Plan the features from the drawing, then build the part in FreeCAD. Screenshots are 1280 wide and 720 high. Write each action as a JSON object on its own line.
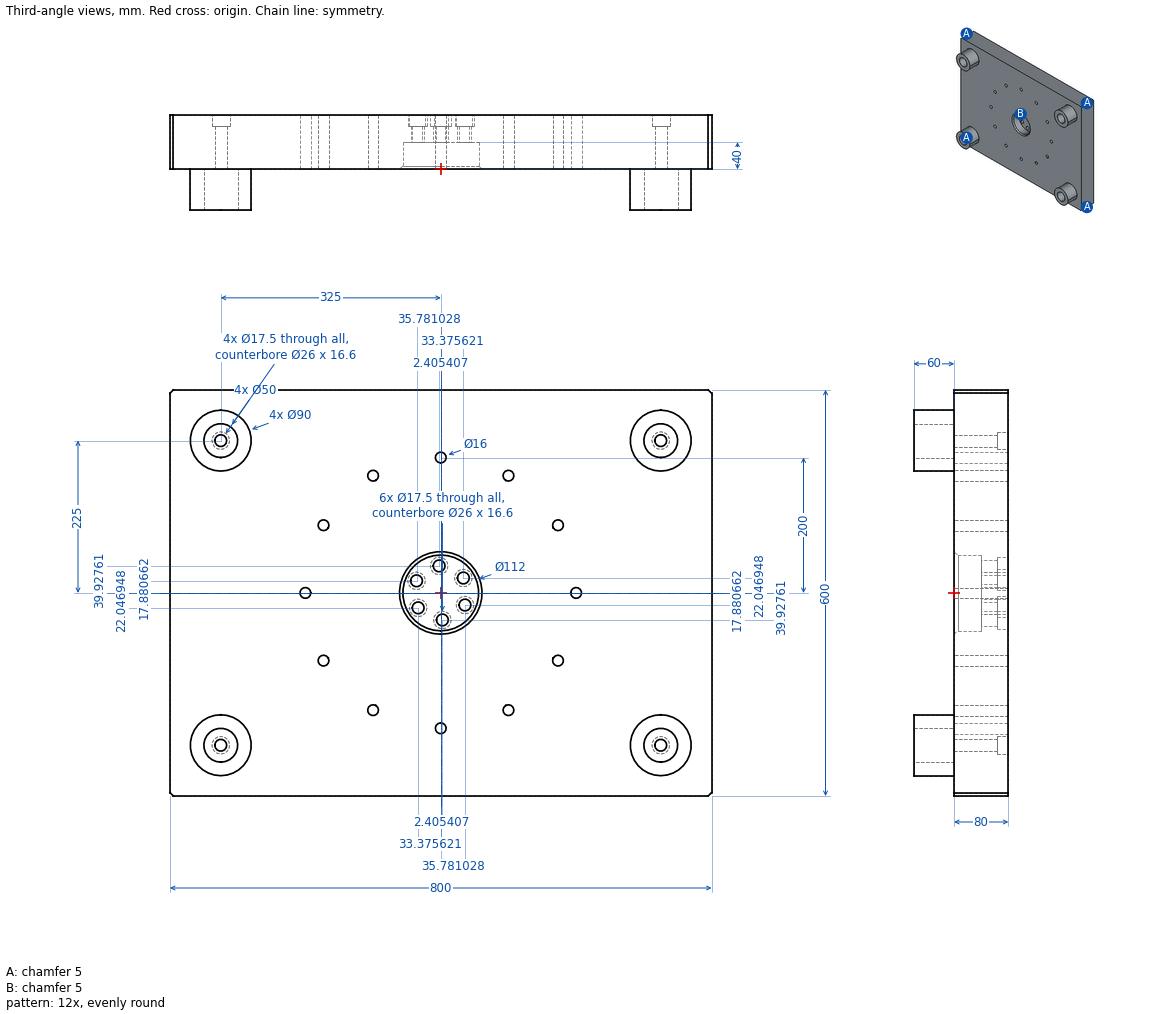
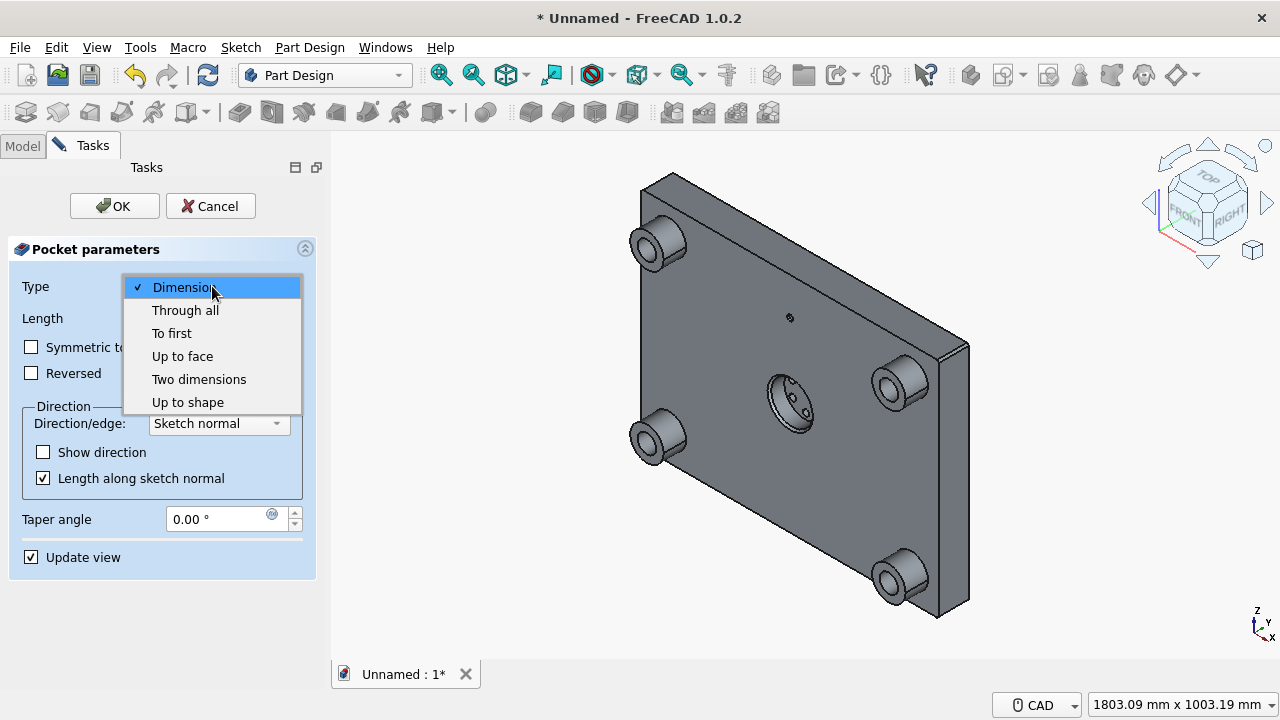
{"action": "left_click", "coordinate": [212, 310]}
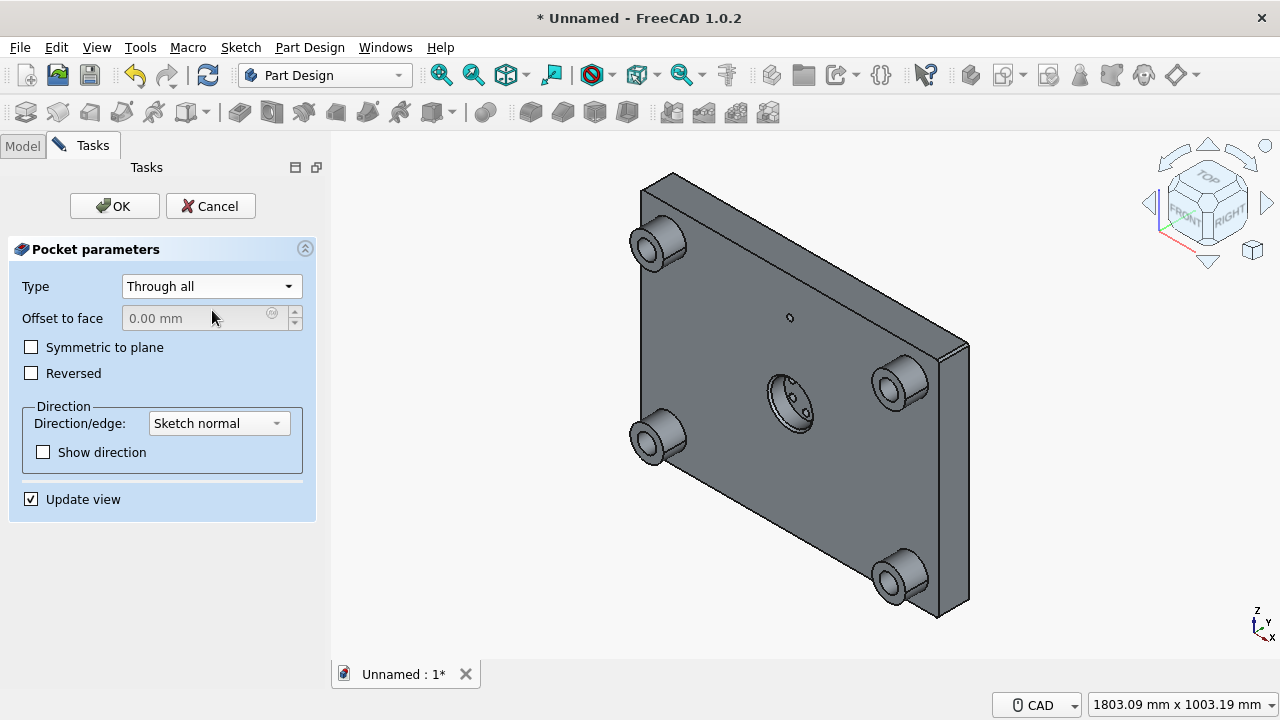
{"action": "left_click", "coordinate": [115, 206]}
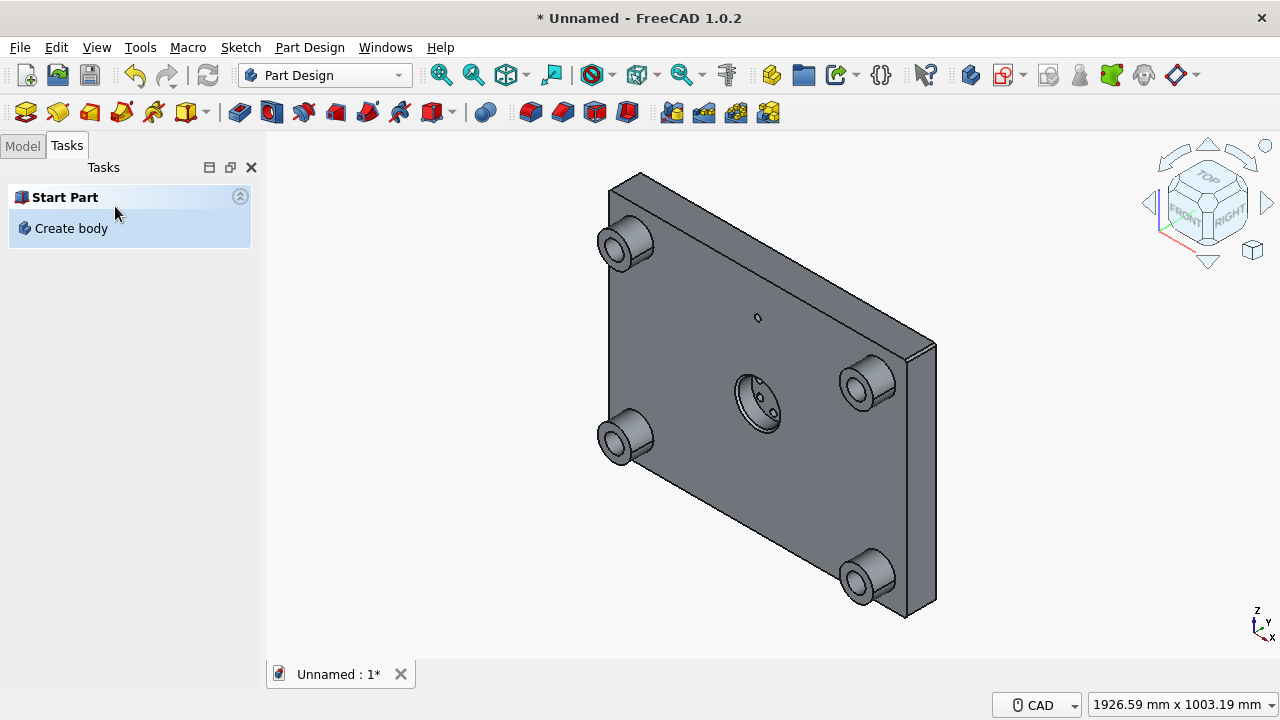
{"action": "left_click", "coordinate": [23, 145]}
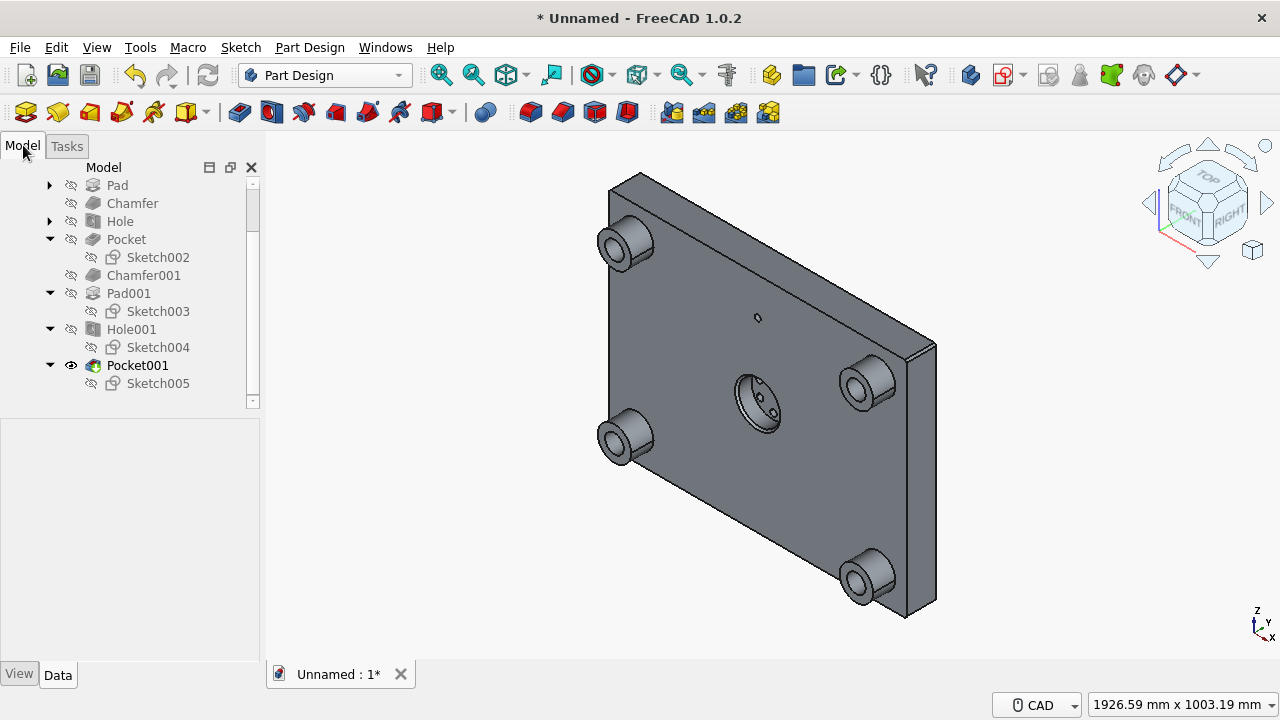
{"action": "left_click", "coordinate": [116, 365]}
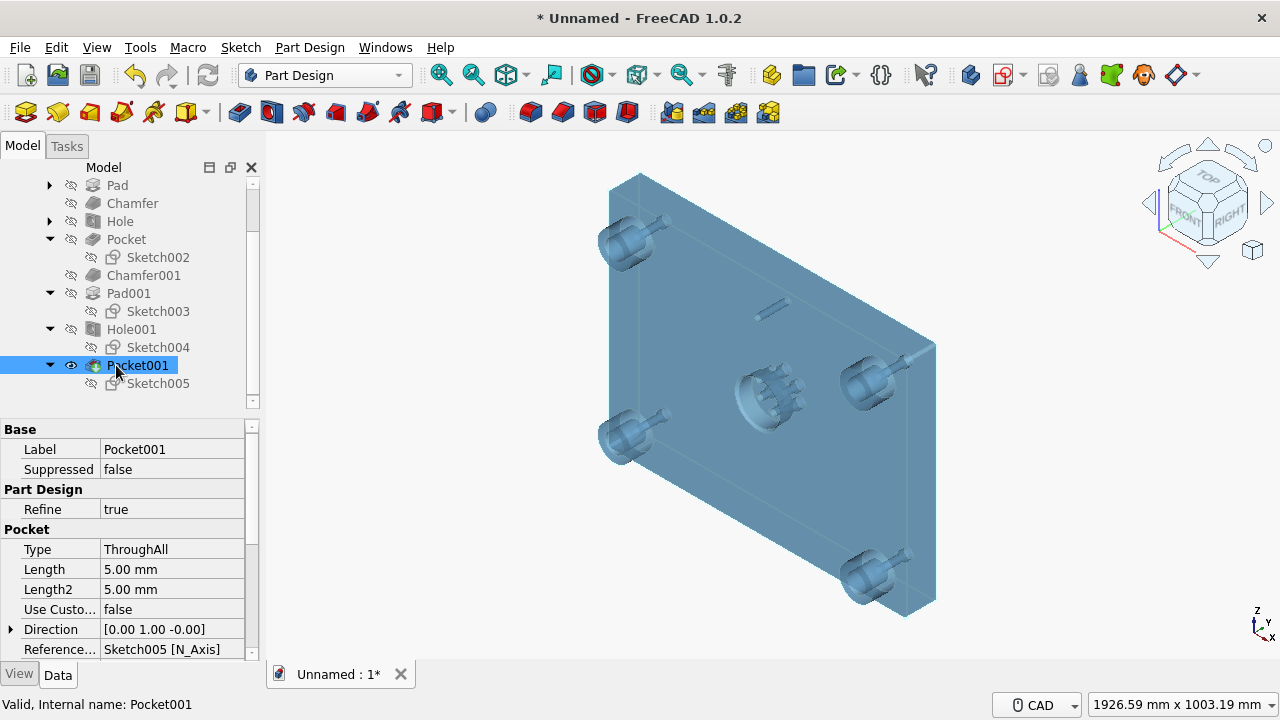
{"action": "left_click", "coordinate": [736, 112]}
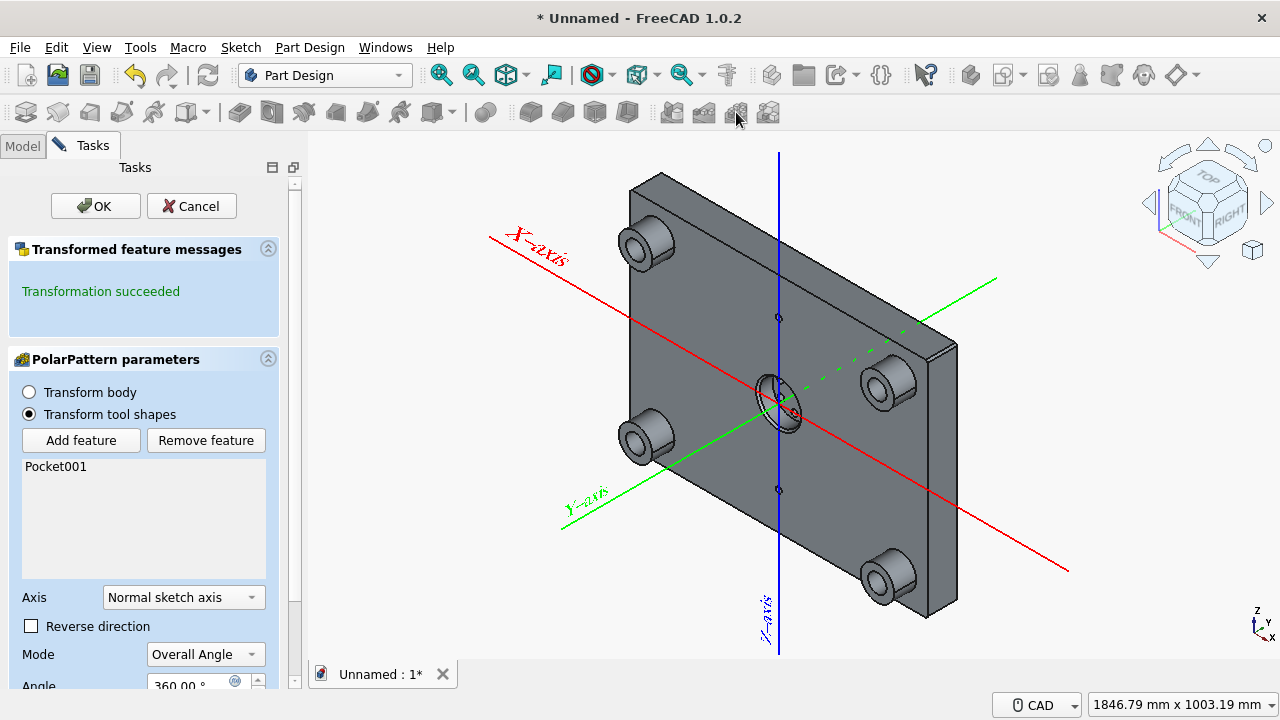
{"action": "left_click", "coordinate": [184, 598]}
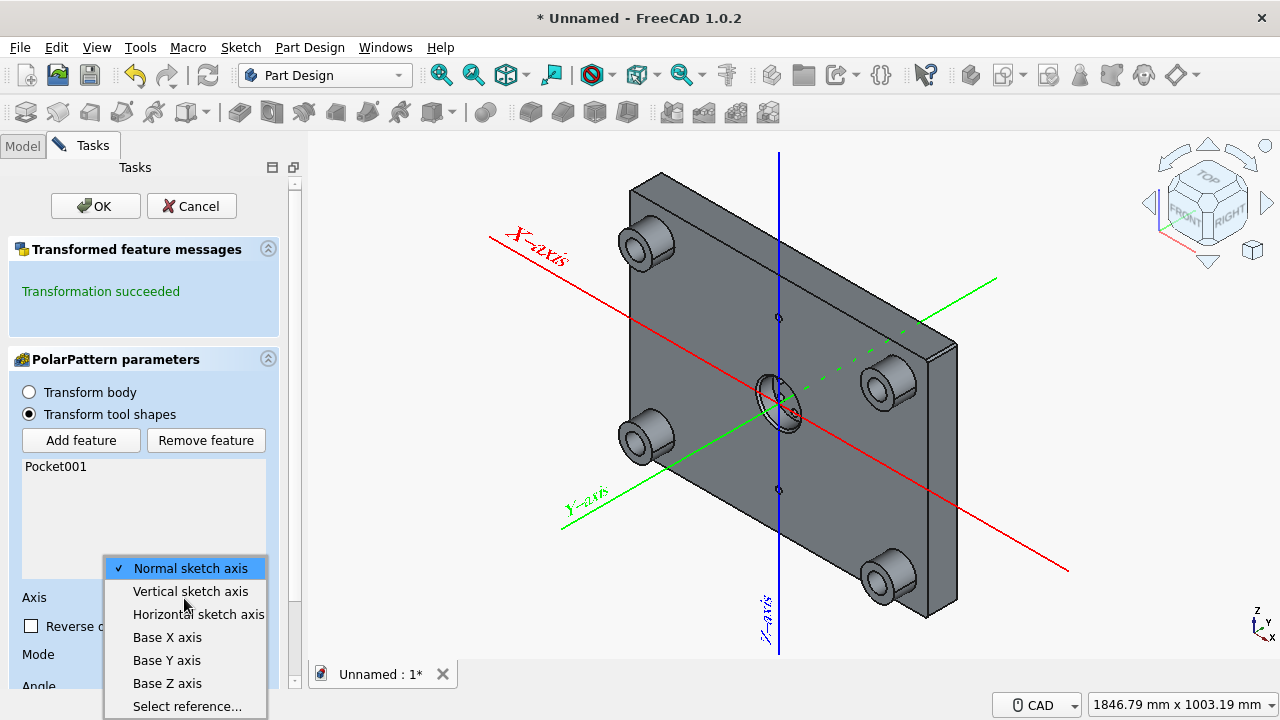
{"action": "left_click", "coordinate": [184, 660]}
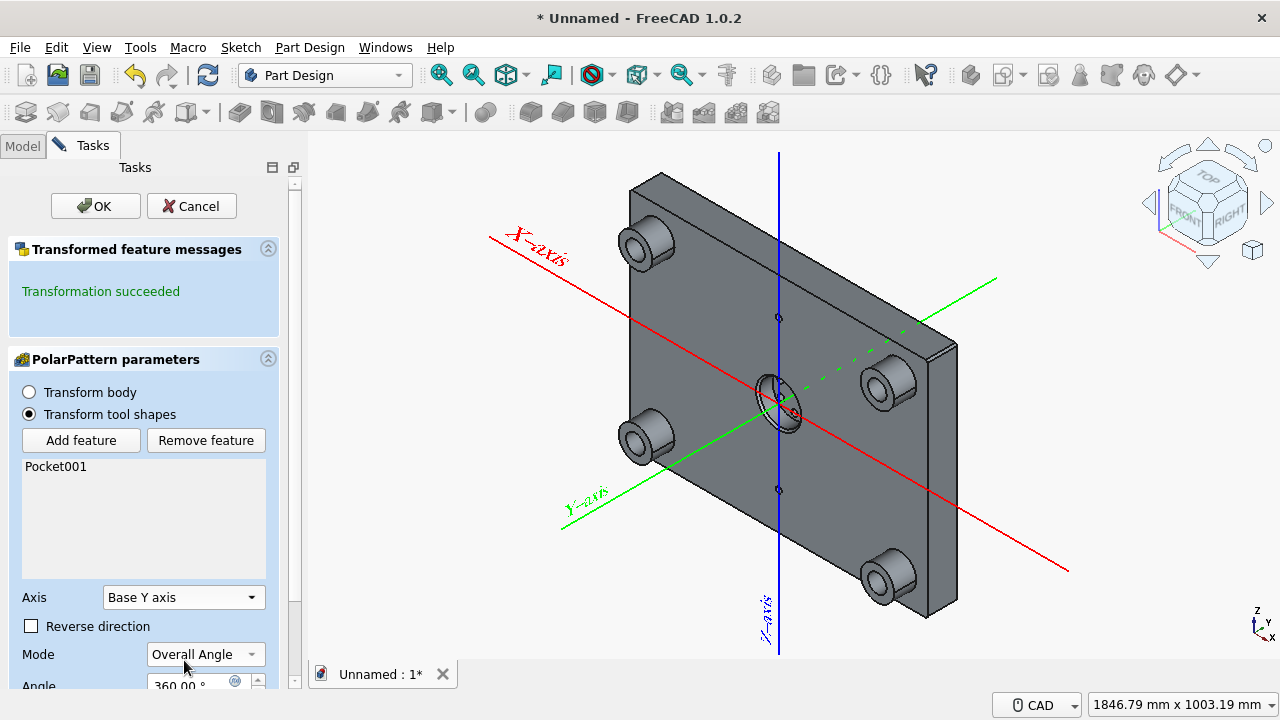
{"action": "scroll", "coordinate": [295, 432], "scroll_direction": "down", "scroll_amount": 2}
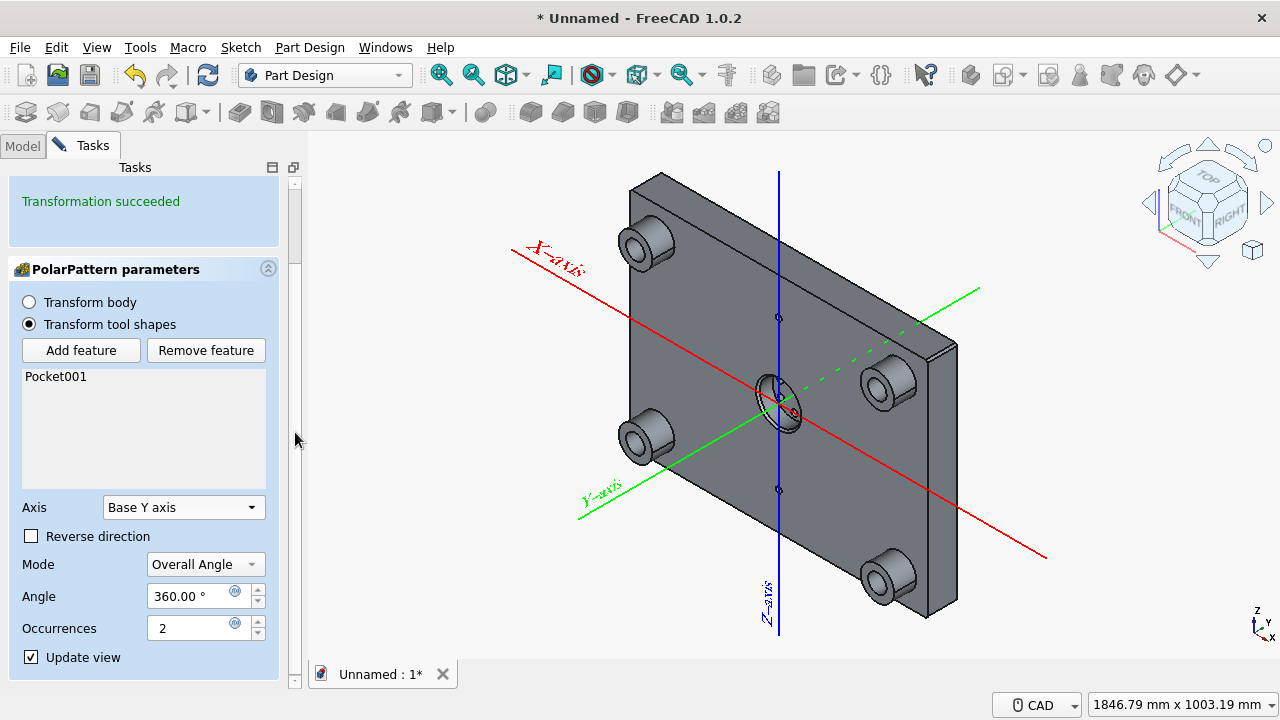
{"action": "triple_click", "coordinate": [198, 628]}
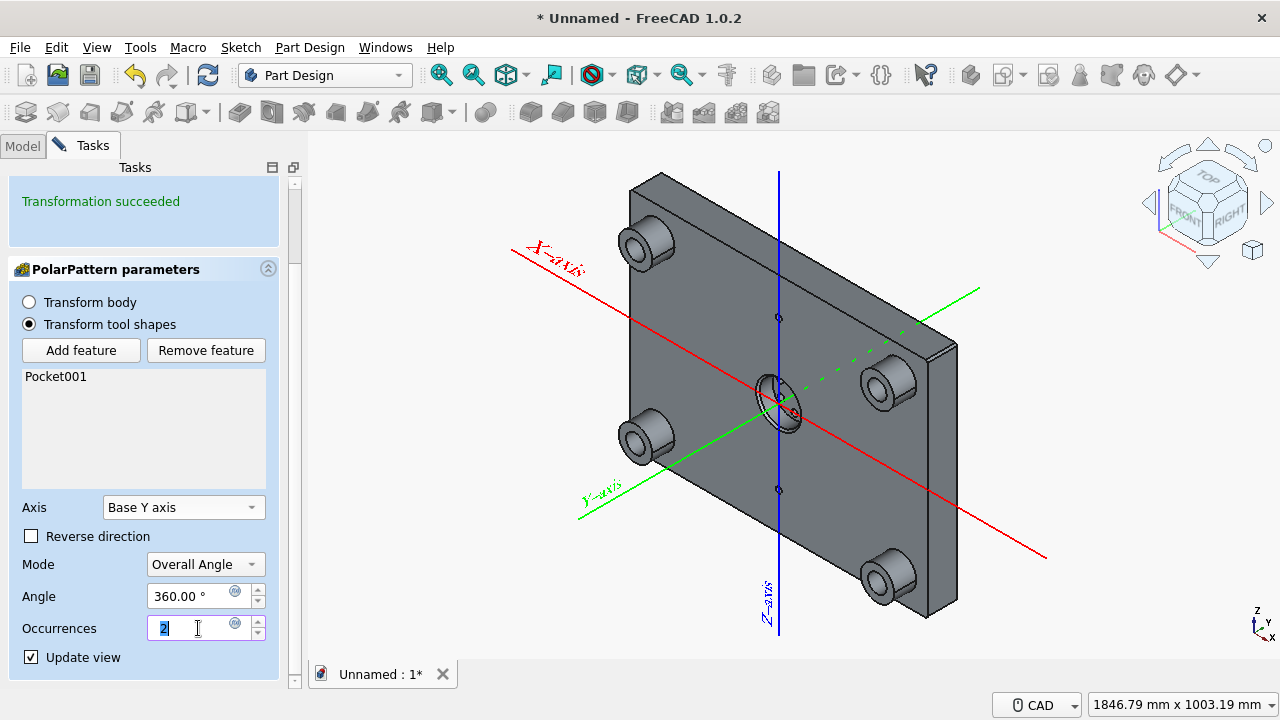
{"action": "type", "text": "12"}
{"action": "key", "text": "Tab"}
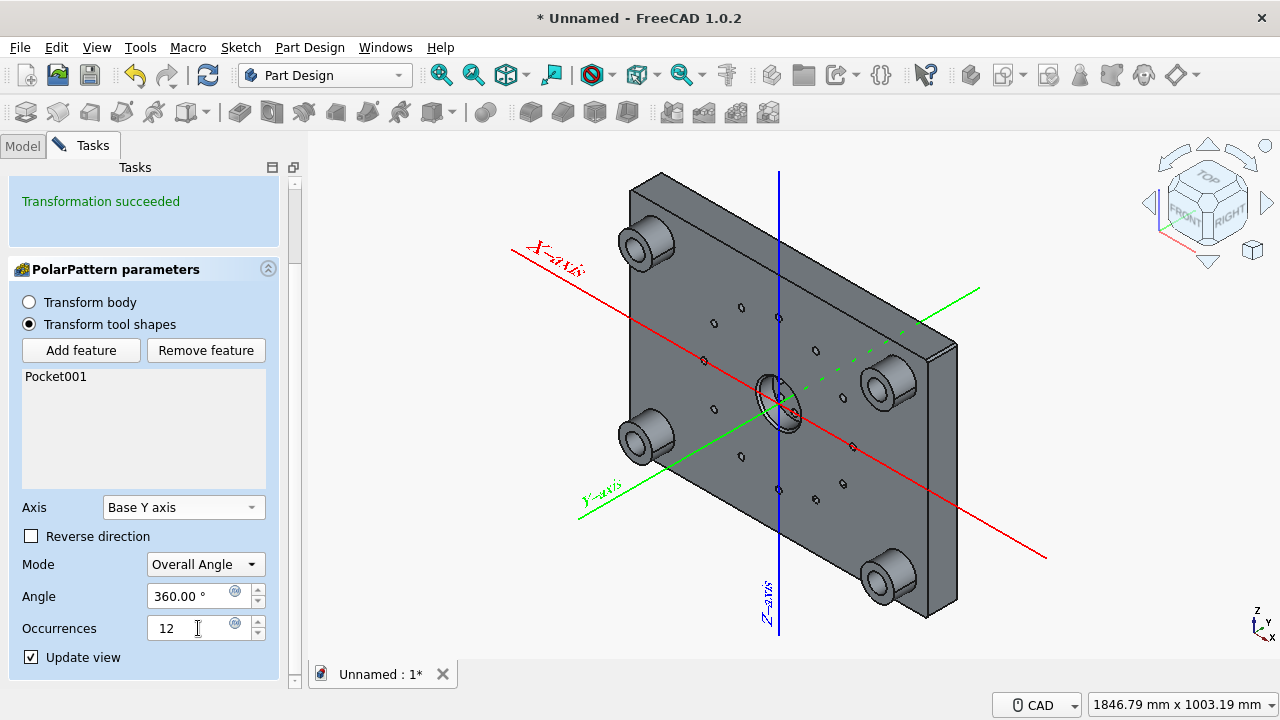
{"action": "scroll", "coordinate": [295, 432], "scroll_direction": "up", "scroll_amount": 3}